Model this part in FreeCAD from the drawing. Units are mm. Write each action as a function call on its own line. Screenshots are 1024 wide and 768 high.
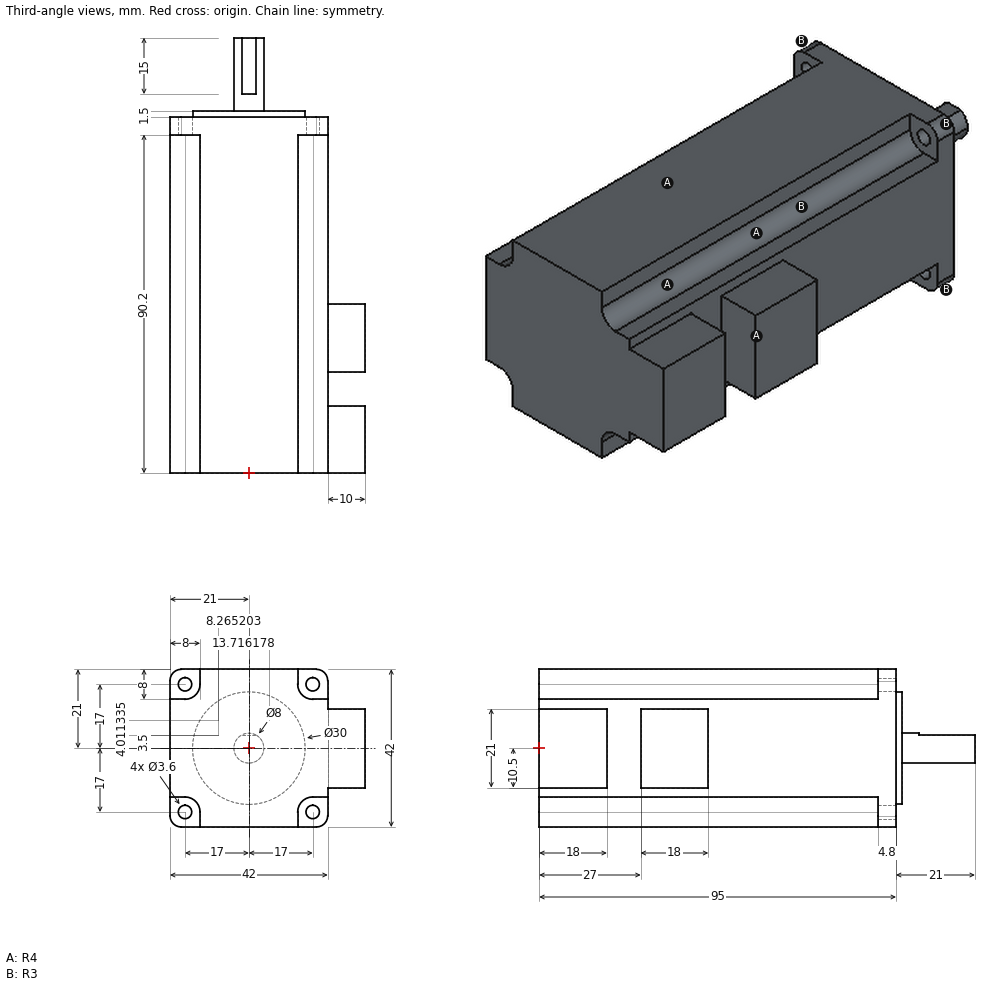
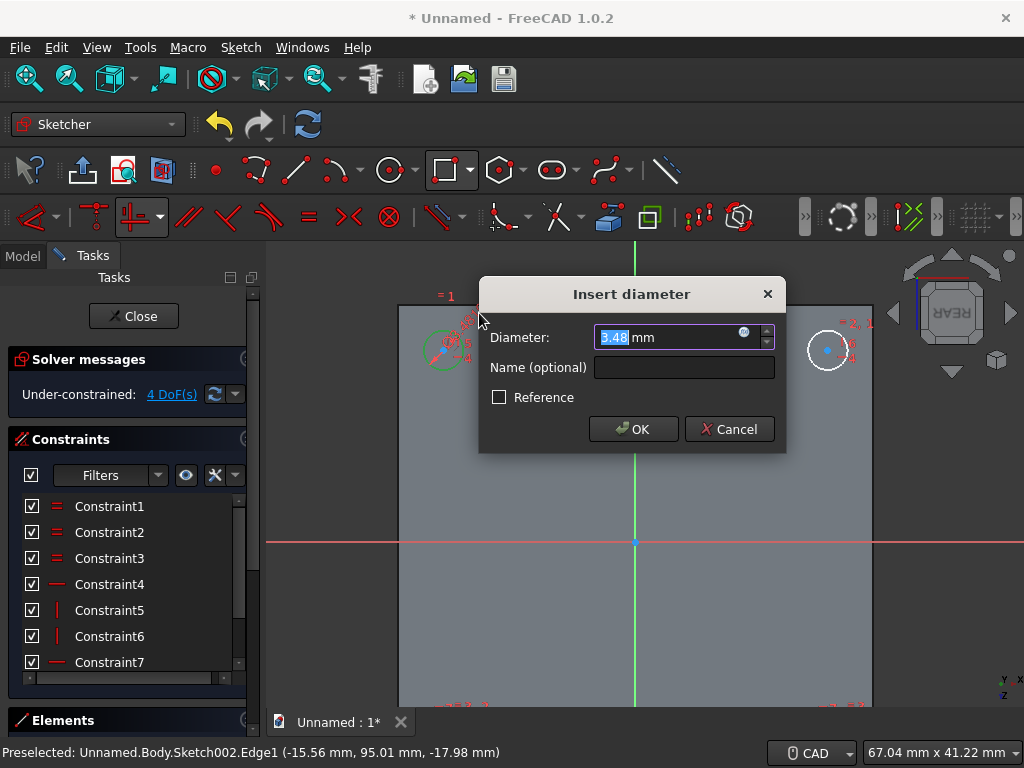
text(3.6)
key(Return)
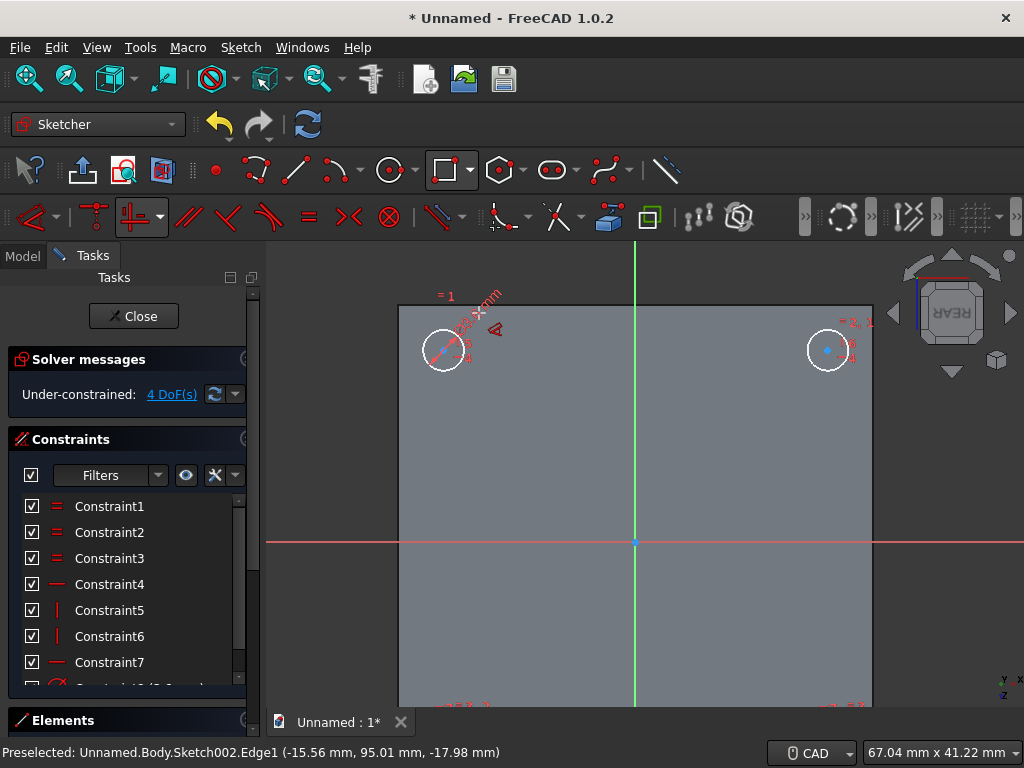
click(444, 350)
click(584, 316)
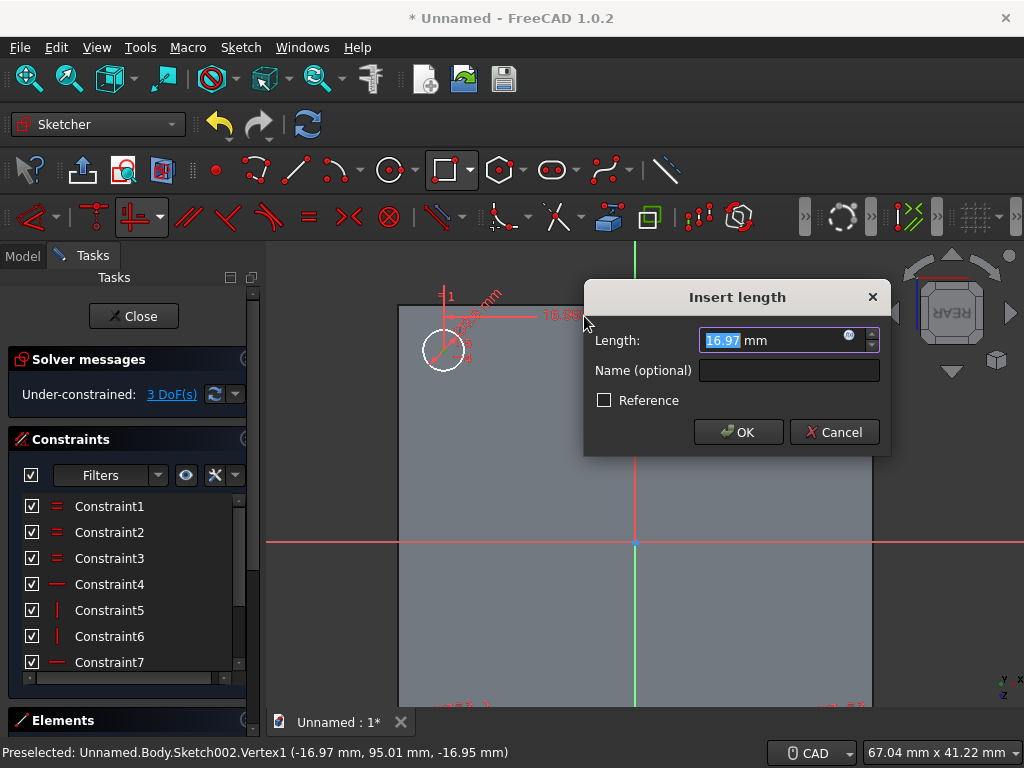
text(17)
key(Return)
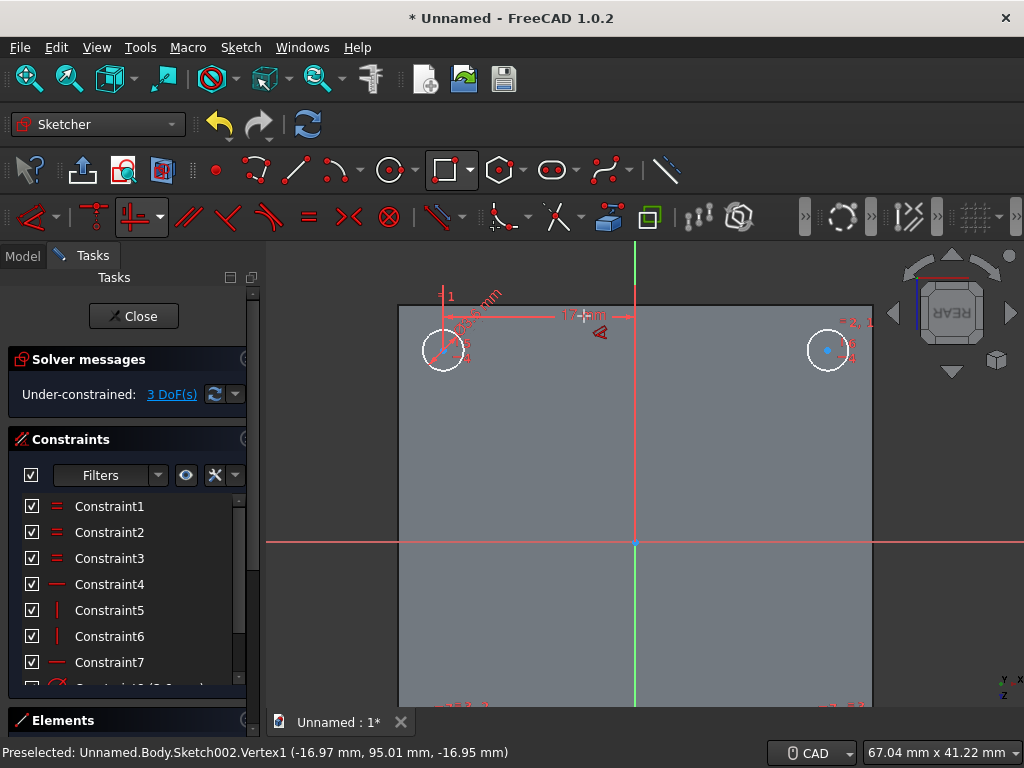
click(443, 350)
click(409, 446)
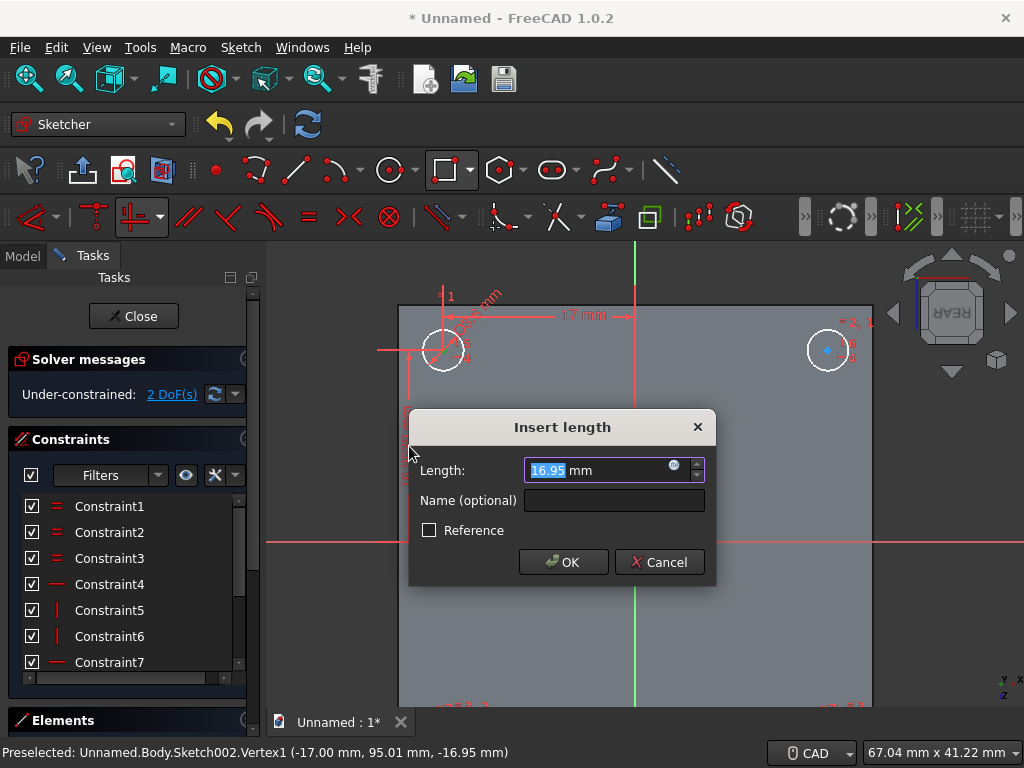
text(17)
key(Return)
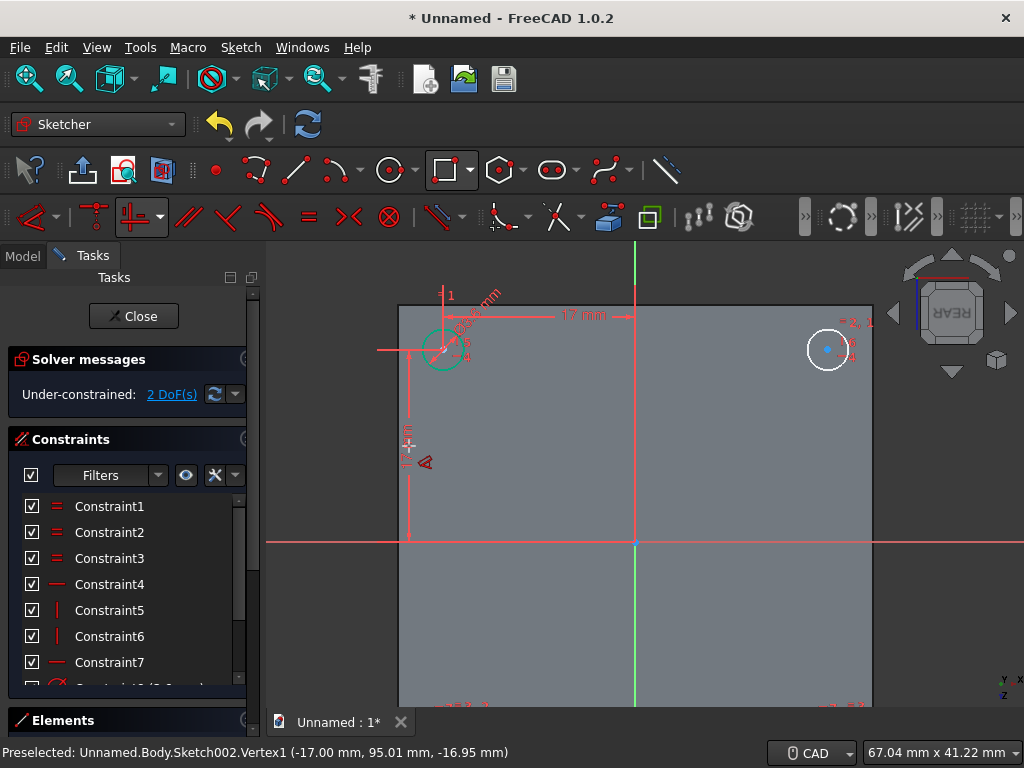
click(828, 350)
click(732, 316)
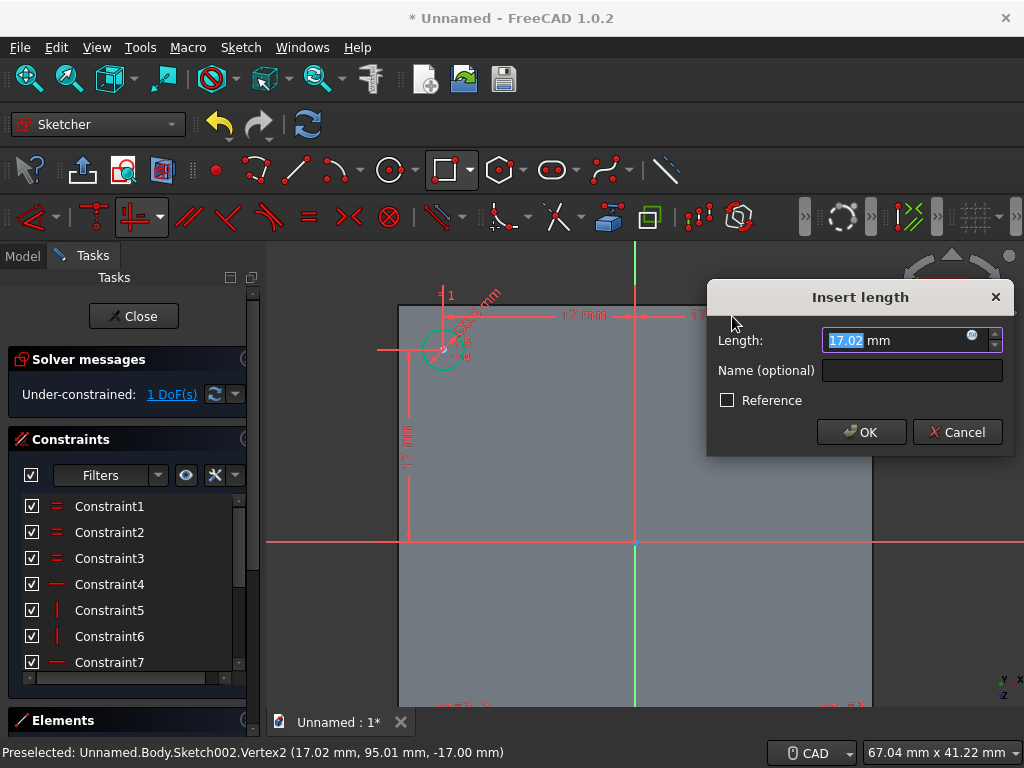
text(17)
key(Return)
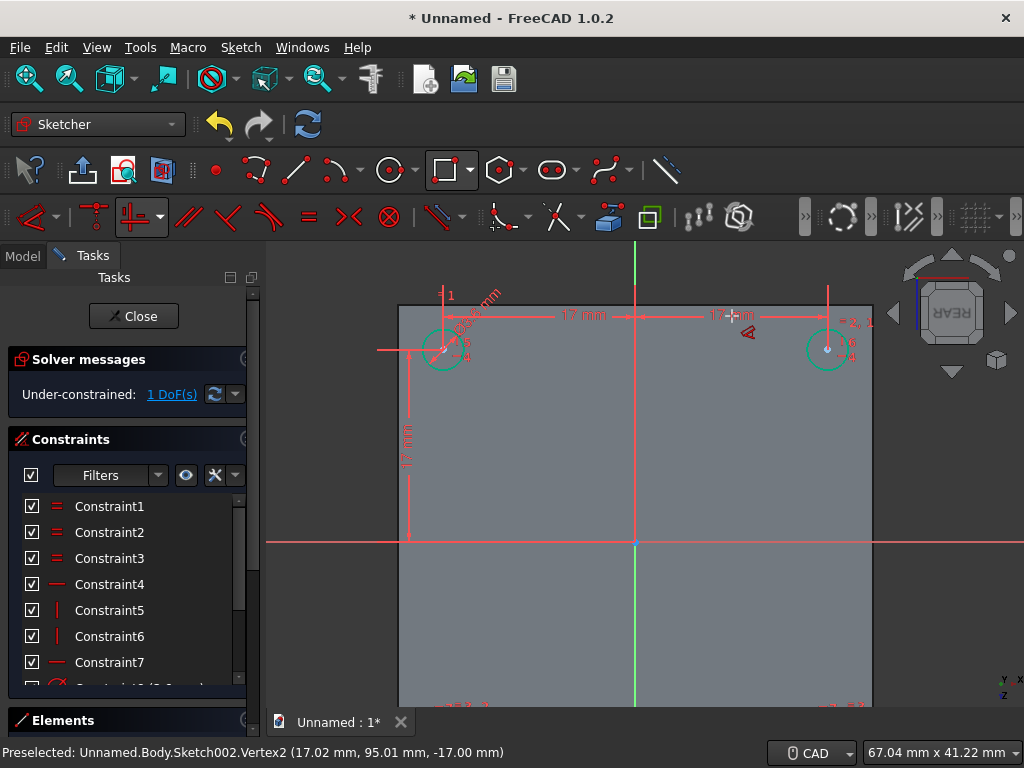
scroll(457, 336, down, 2)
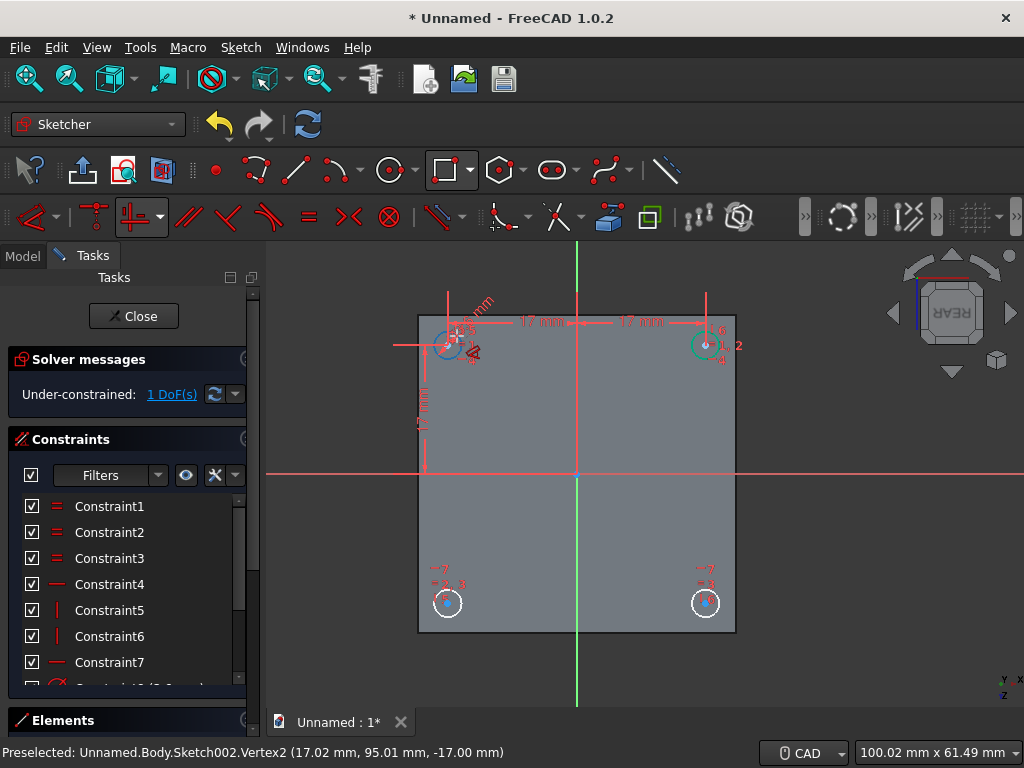
click(448, 603)
click(414, 539)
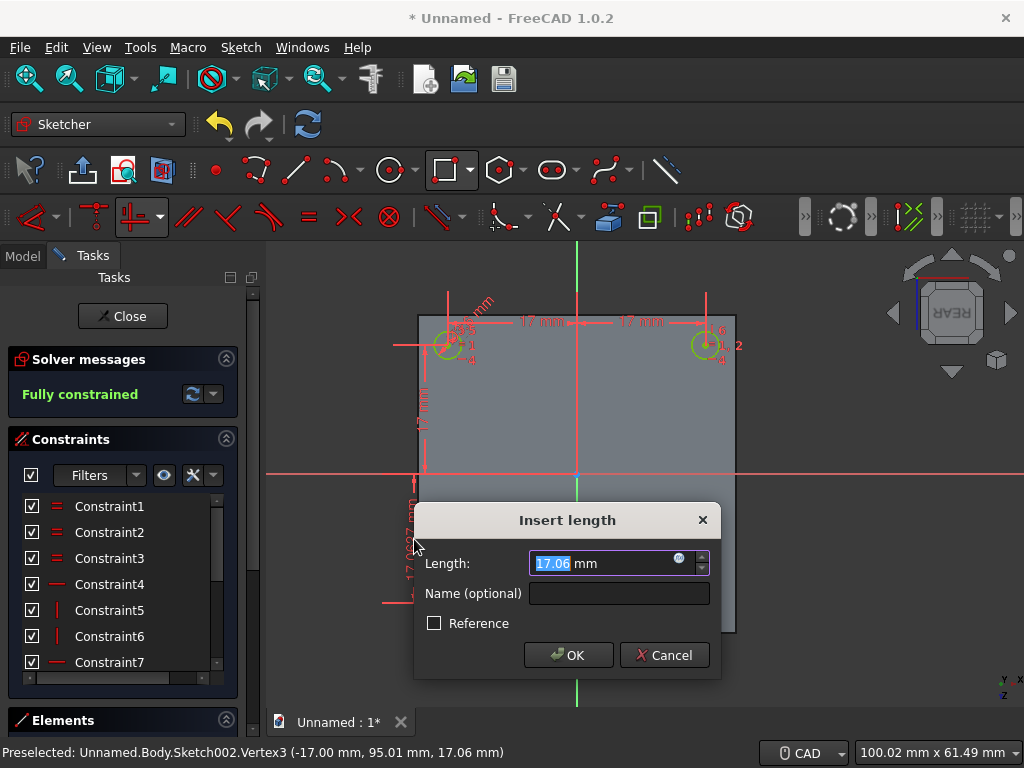
text(17)
key(Return)
key(Escape)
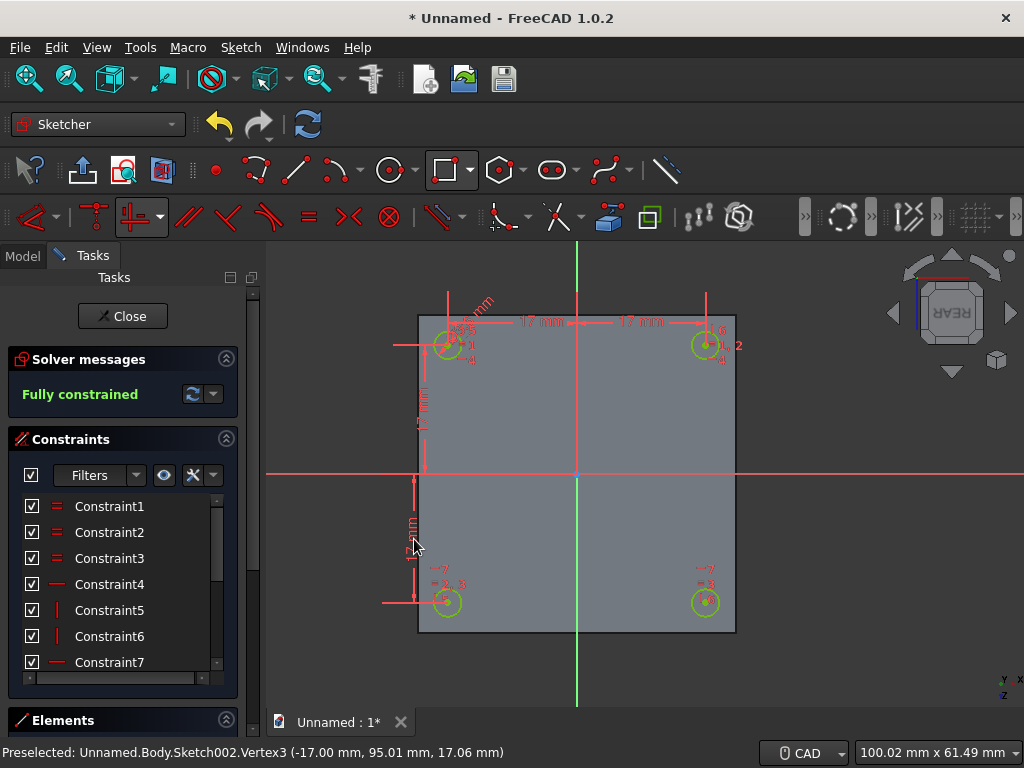
click(123, 316)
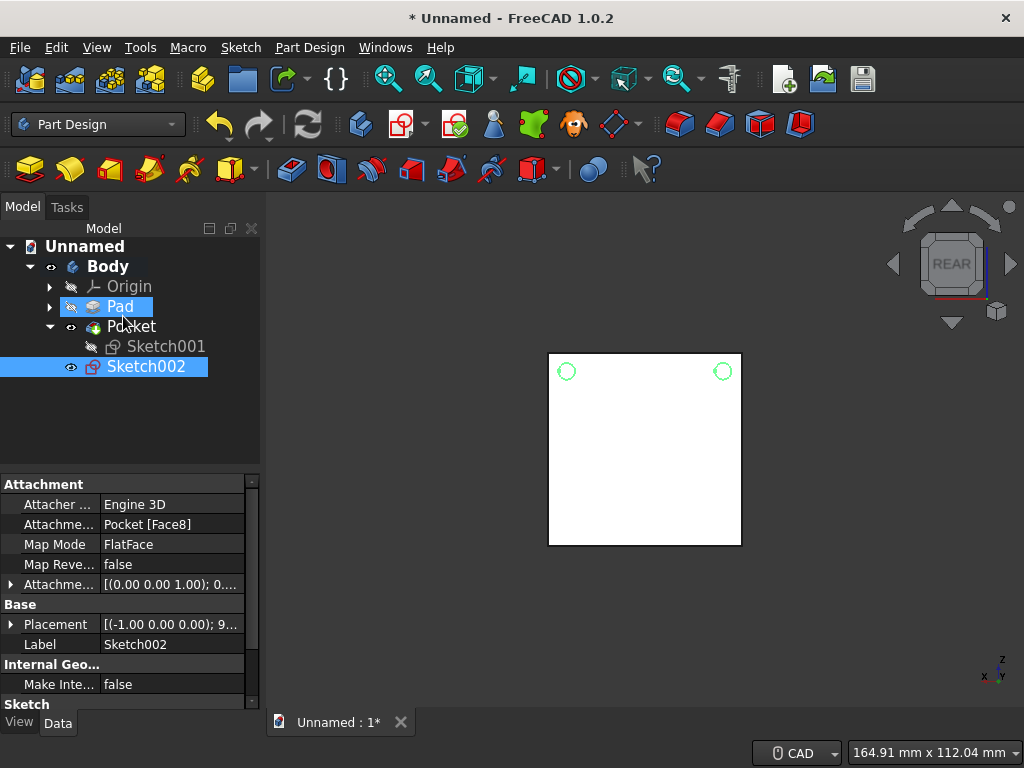
click(292, 170)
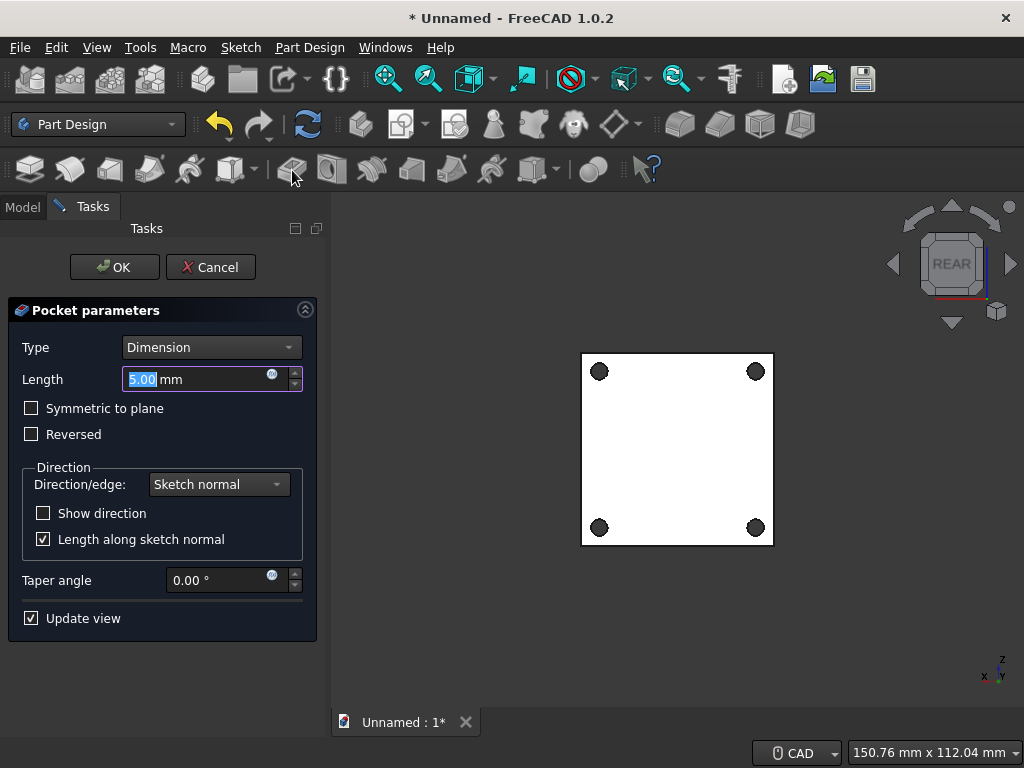
text(4.8)
key(Tab)